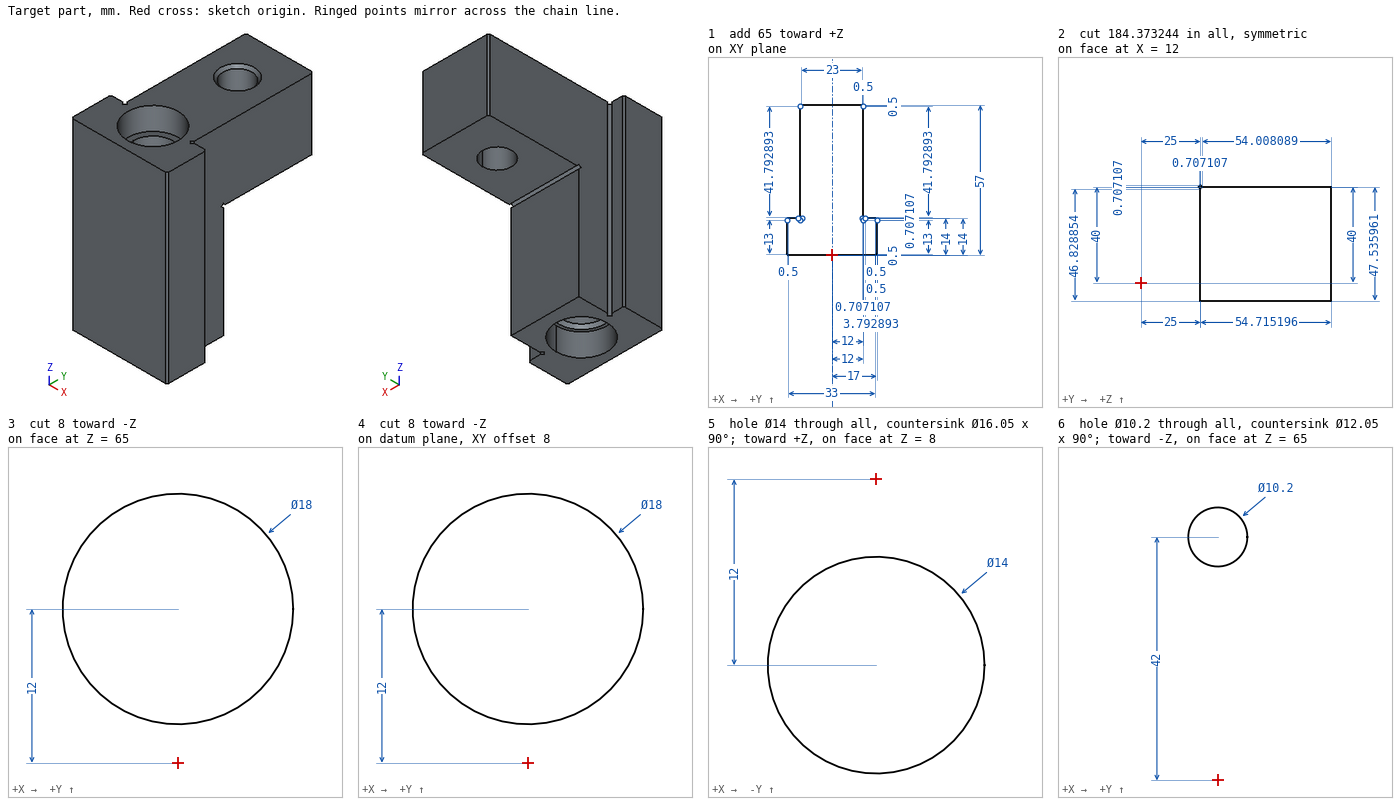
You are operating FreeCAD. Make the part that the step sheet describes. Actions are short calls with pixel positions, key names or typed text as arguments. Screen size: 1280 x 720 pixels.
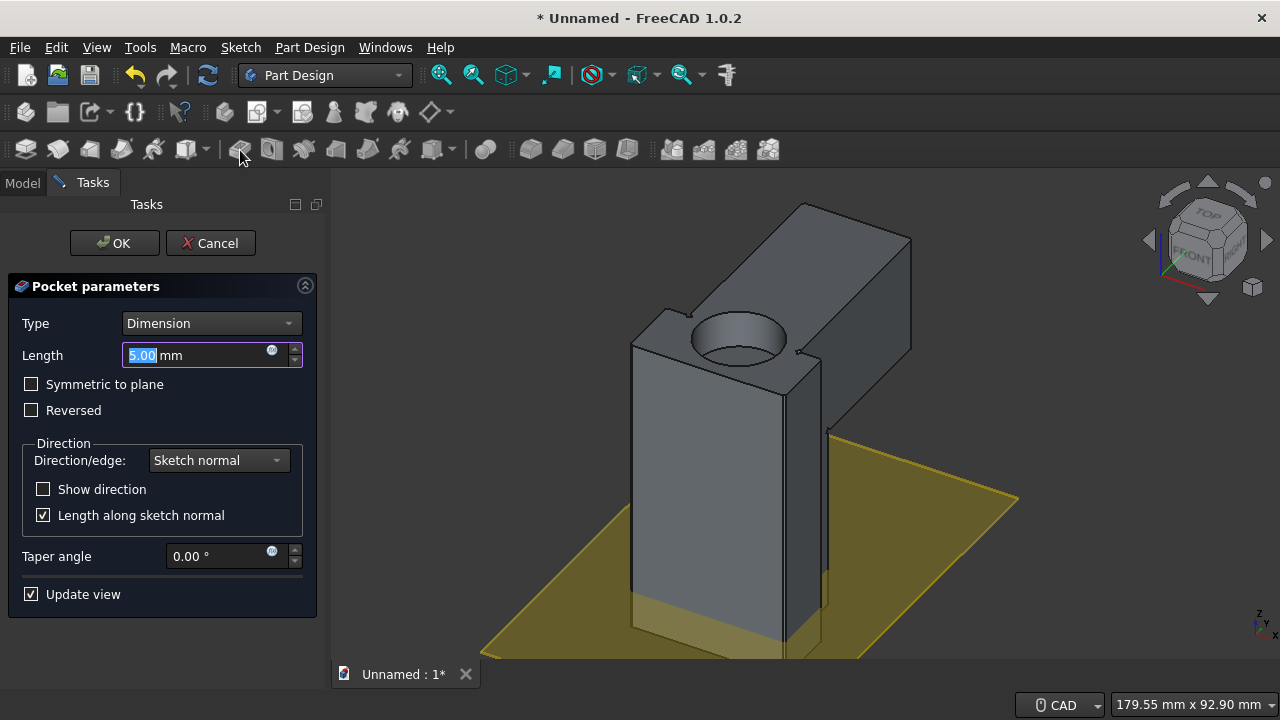
text(8)
key(Tab)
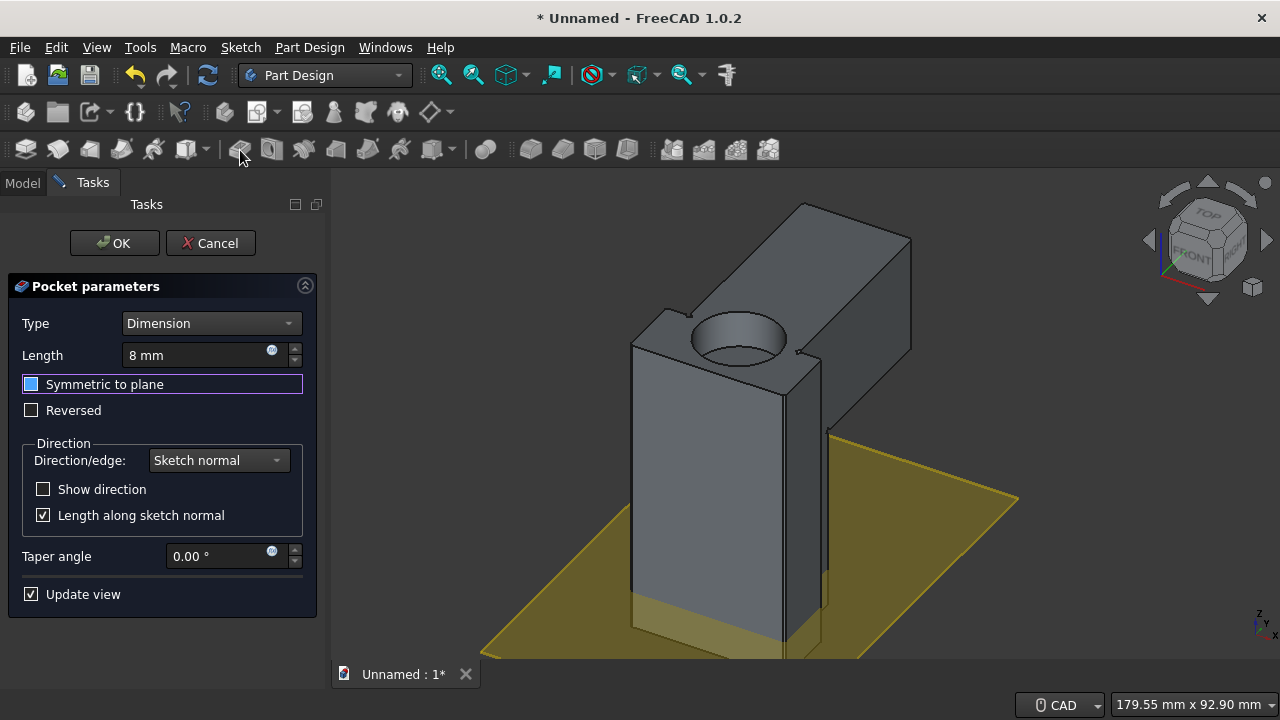
click(115, 243)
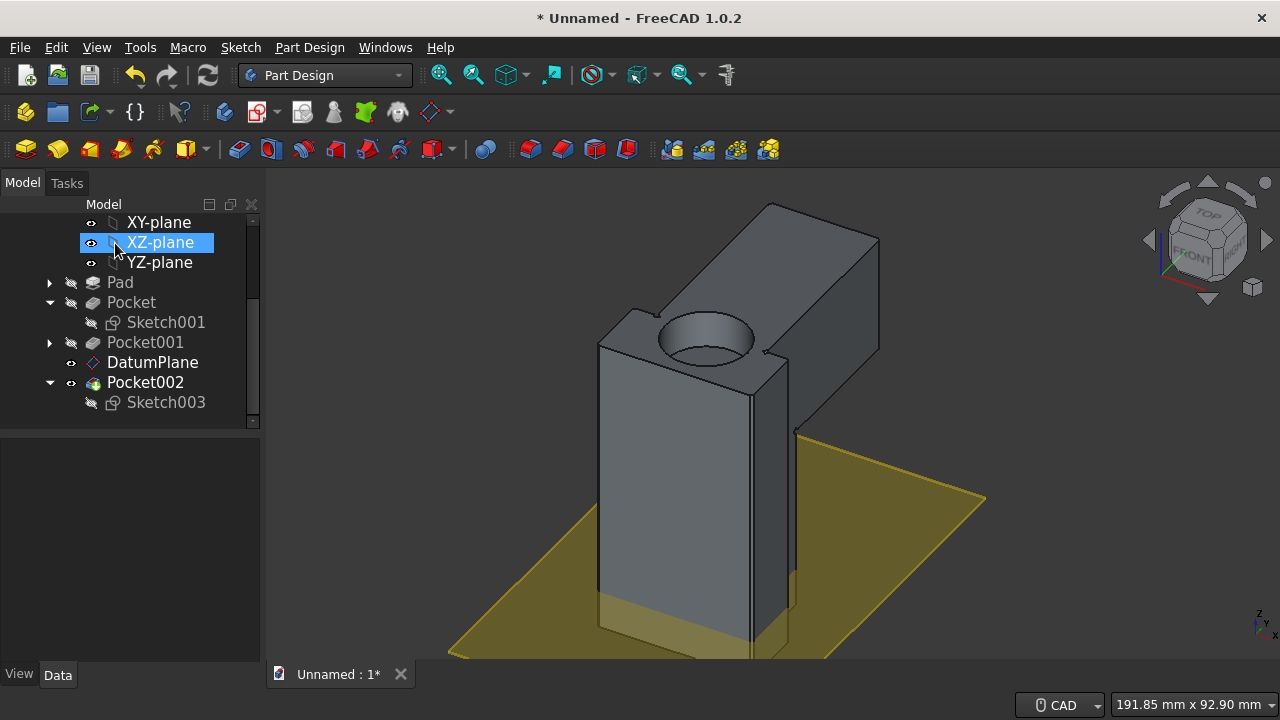
click(116, 363)
key(space)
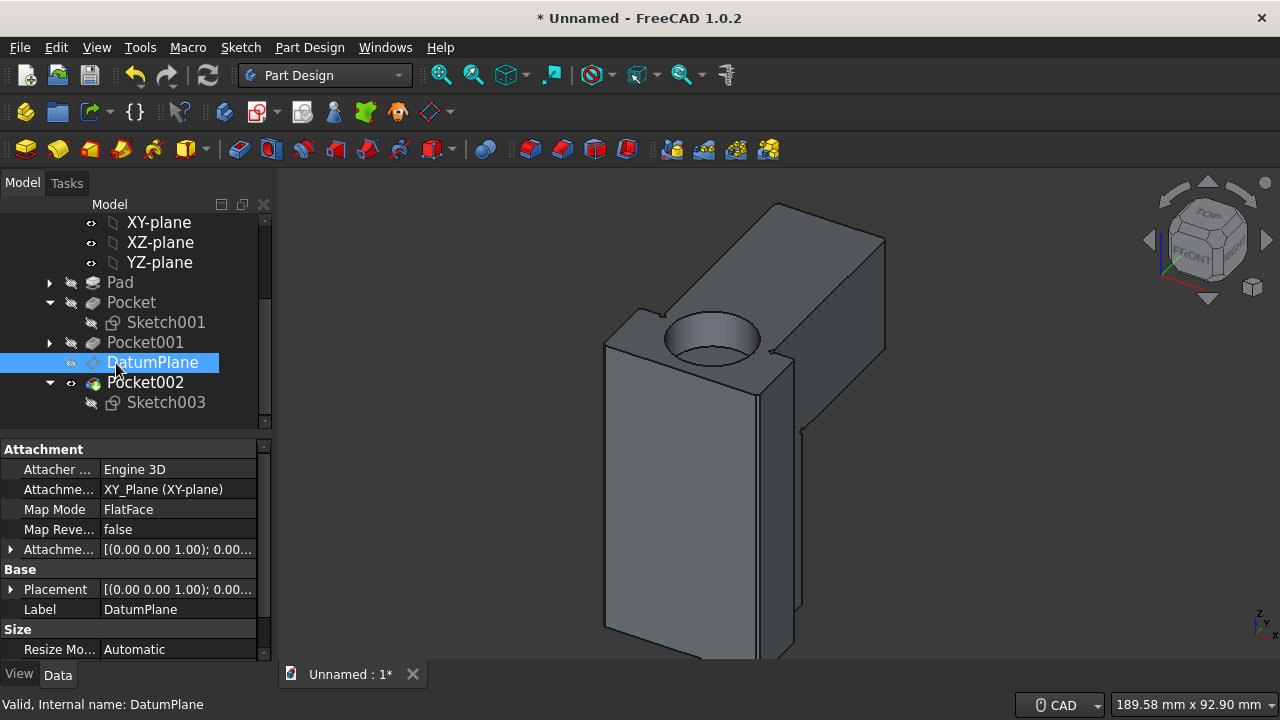
key(v)
key(f)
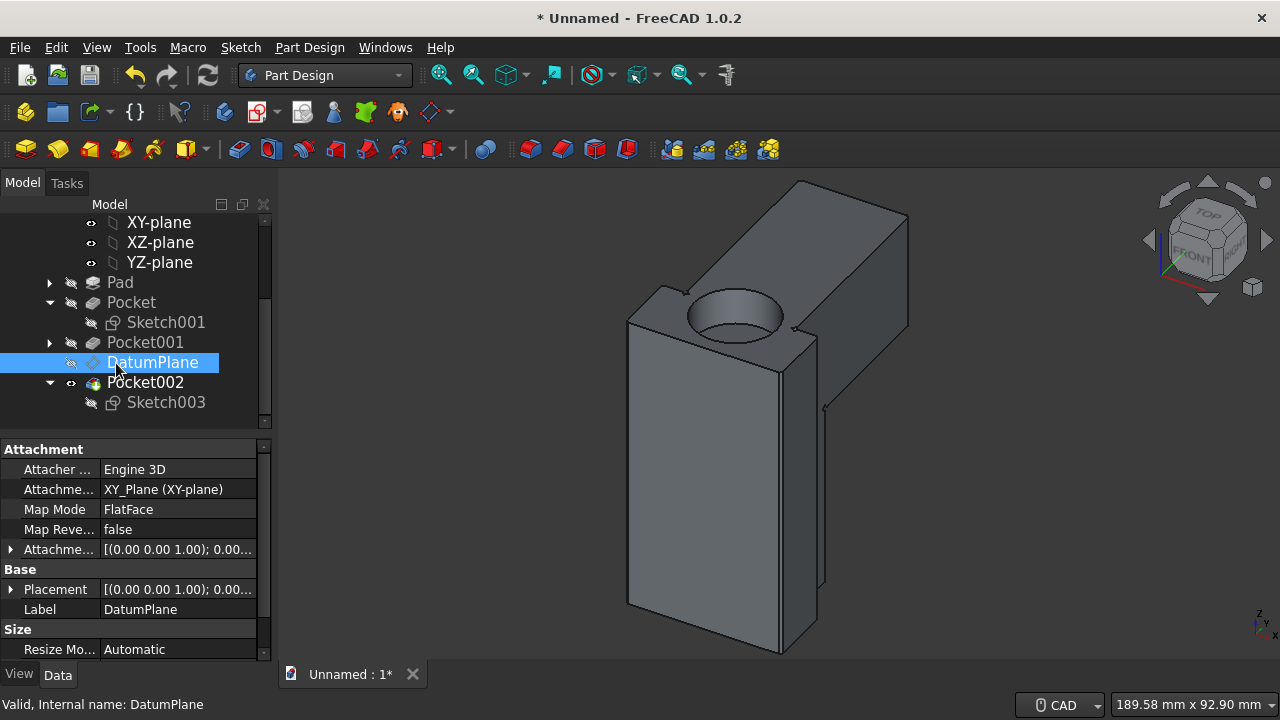
key(5)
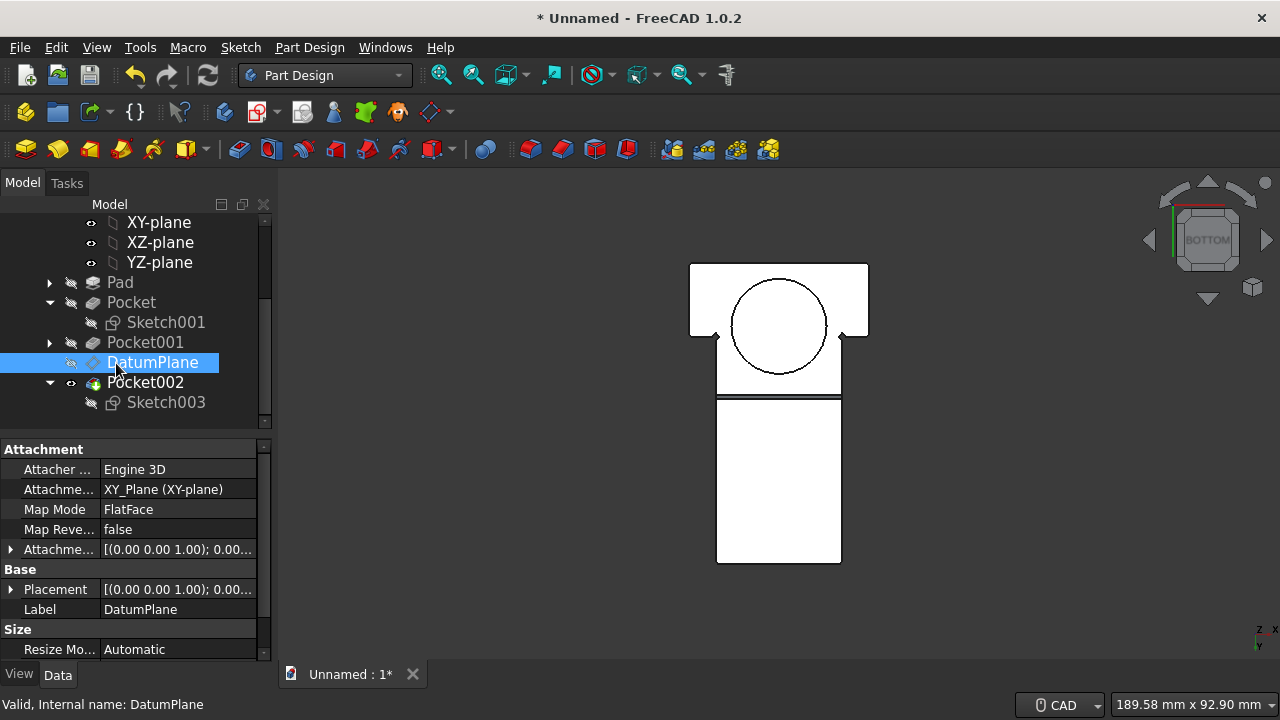
click(779, 325)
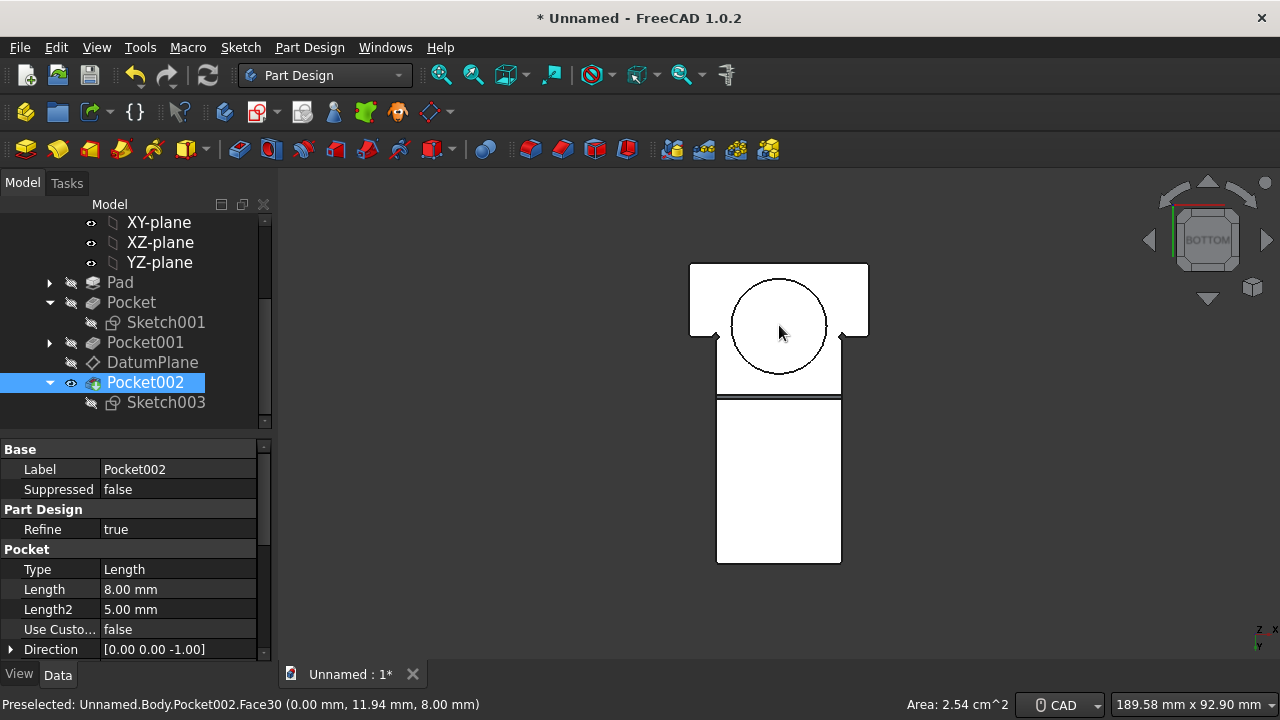
click(258, 112)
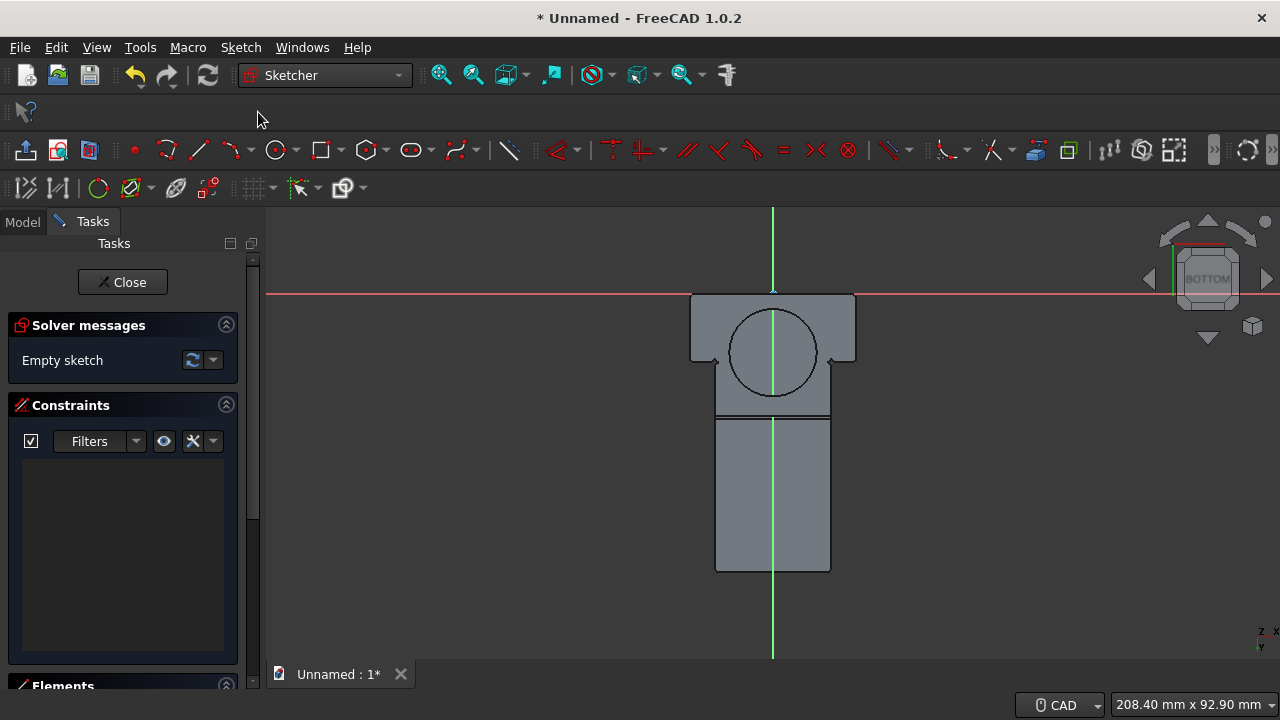
scroll(803, 301, up, 6)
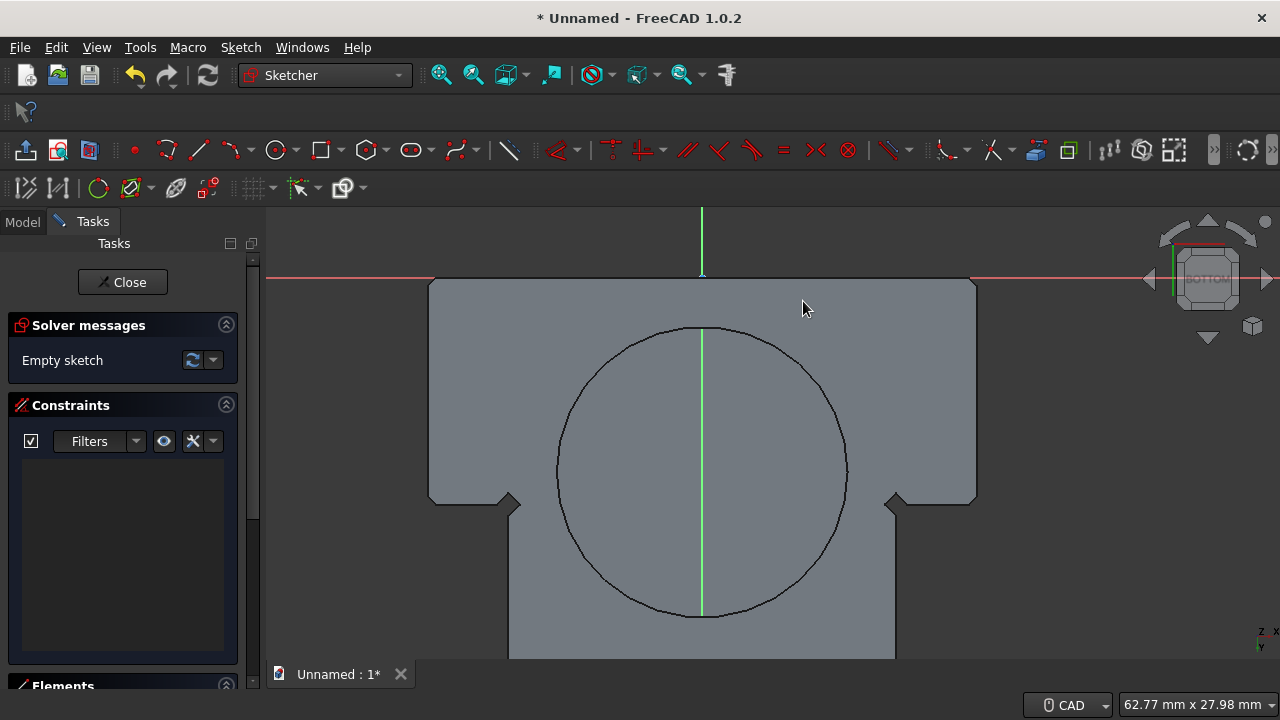
key(g)
key(c)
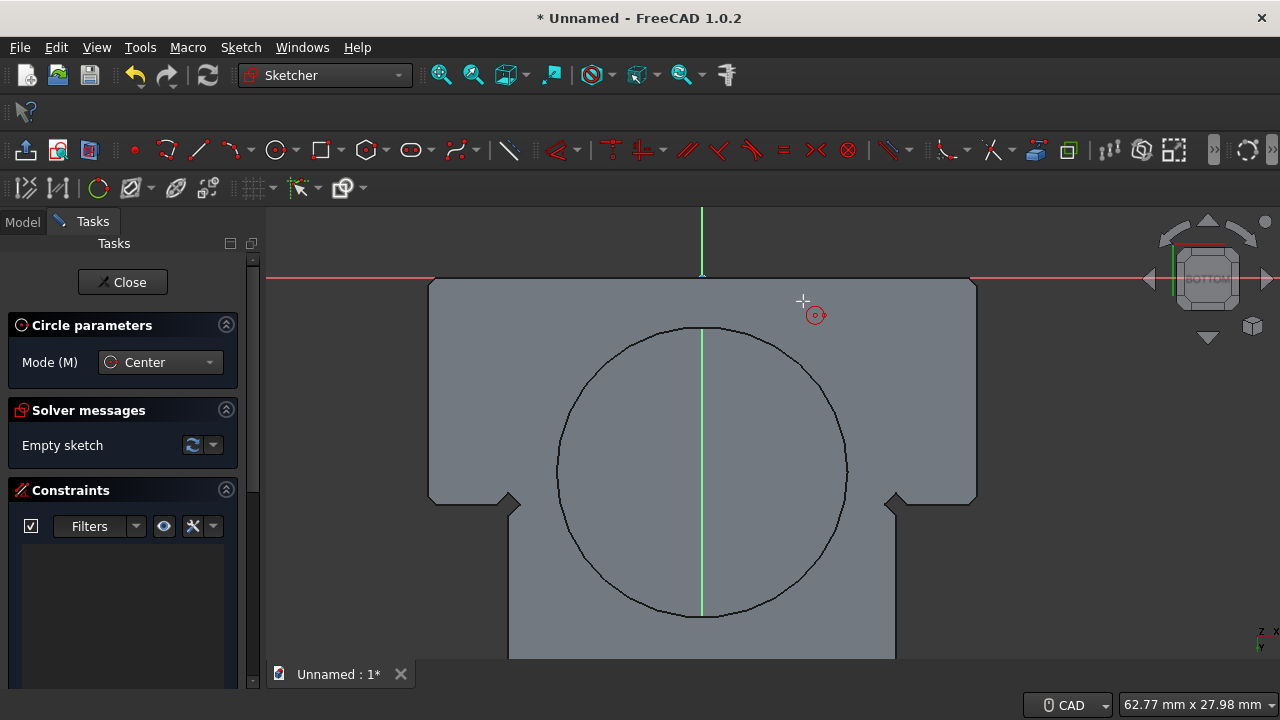
click(702, 472)
click(782, 392)
key(Escape)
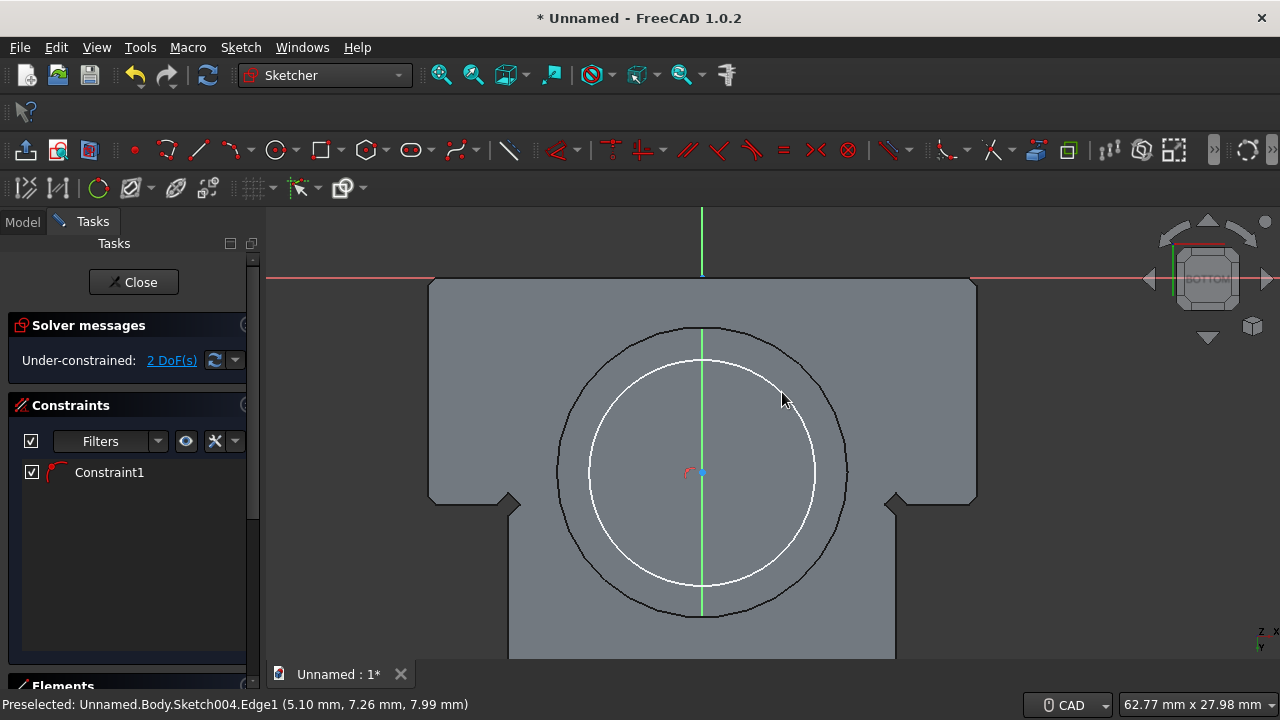
click(556, 150)